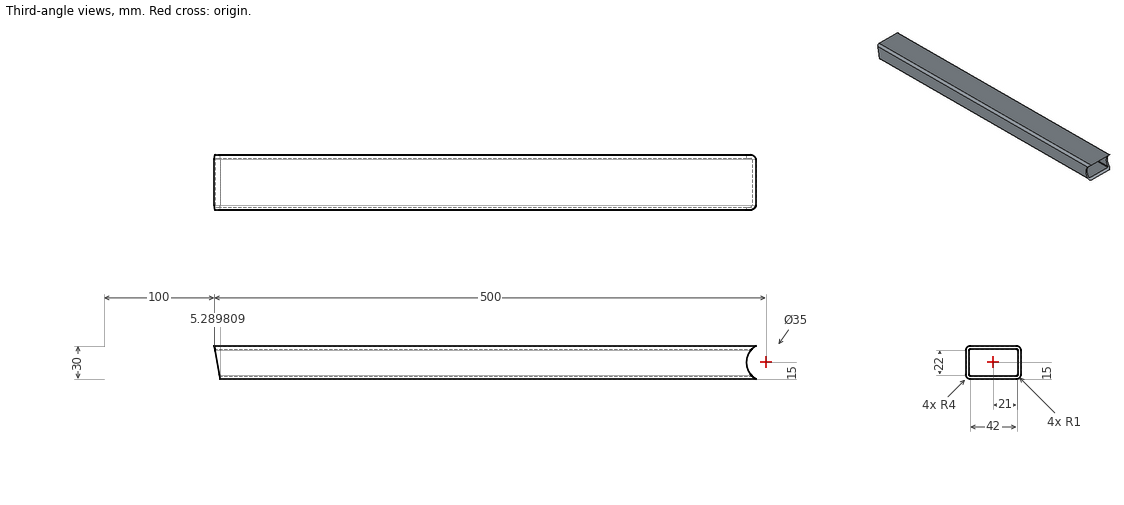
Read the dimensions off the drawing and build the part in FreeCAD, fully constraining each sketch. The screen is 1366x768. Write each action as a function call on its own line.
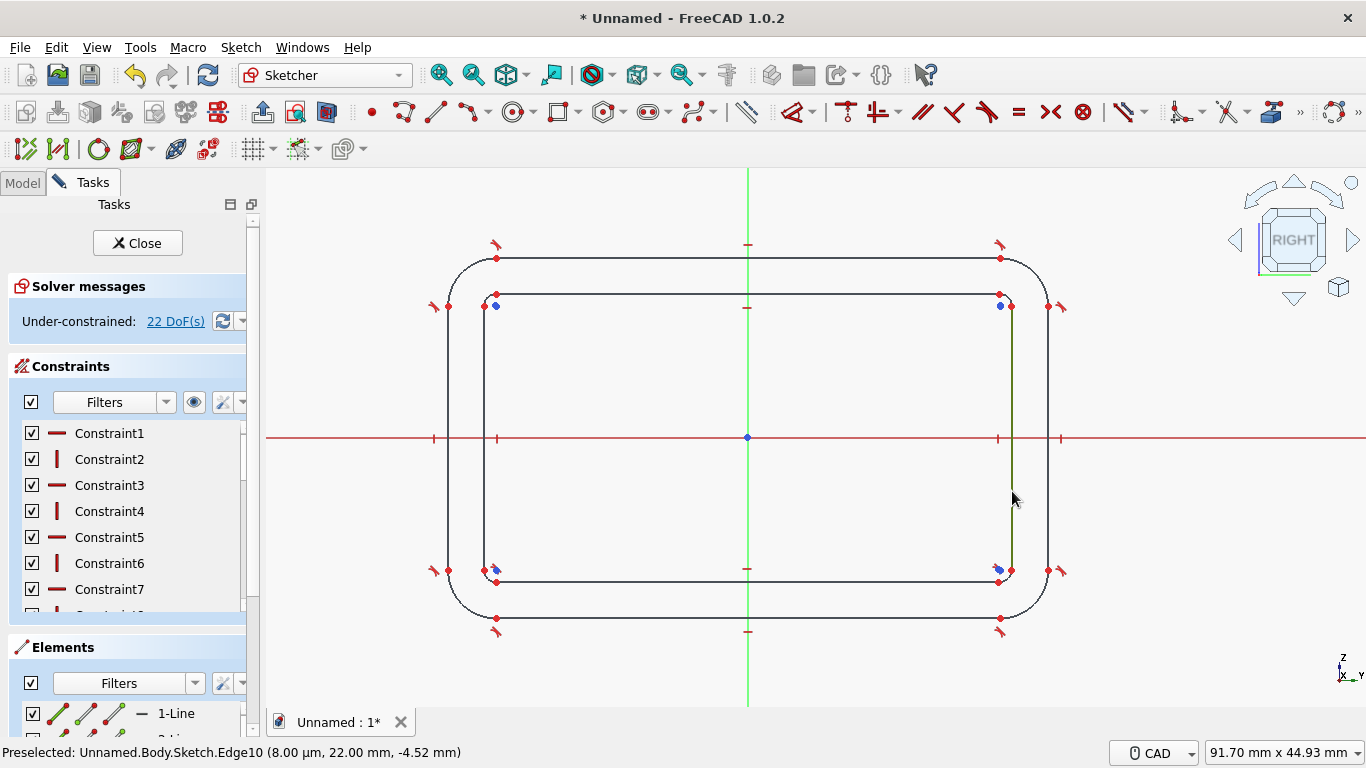
scroll(1008, 579, up, 2)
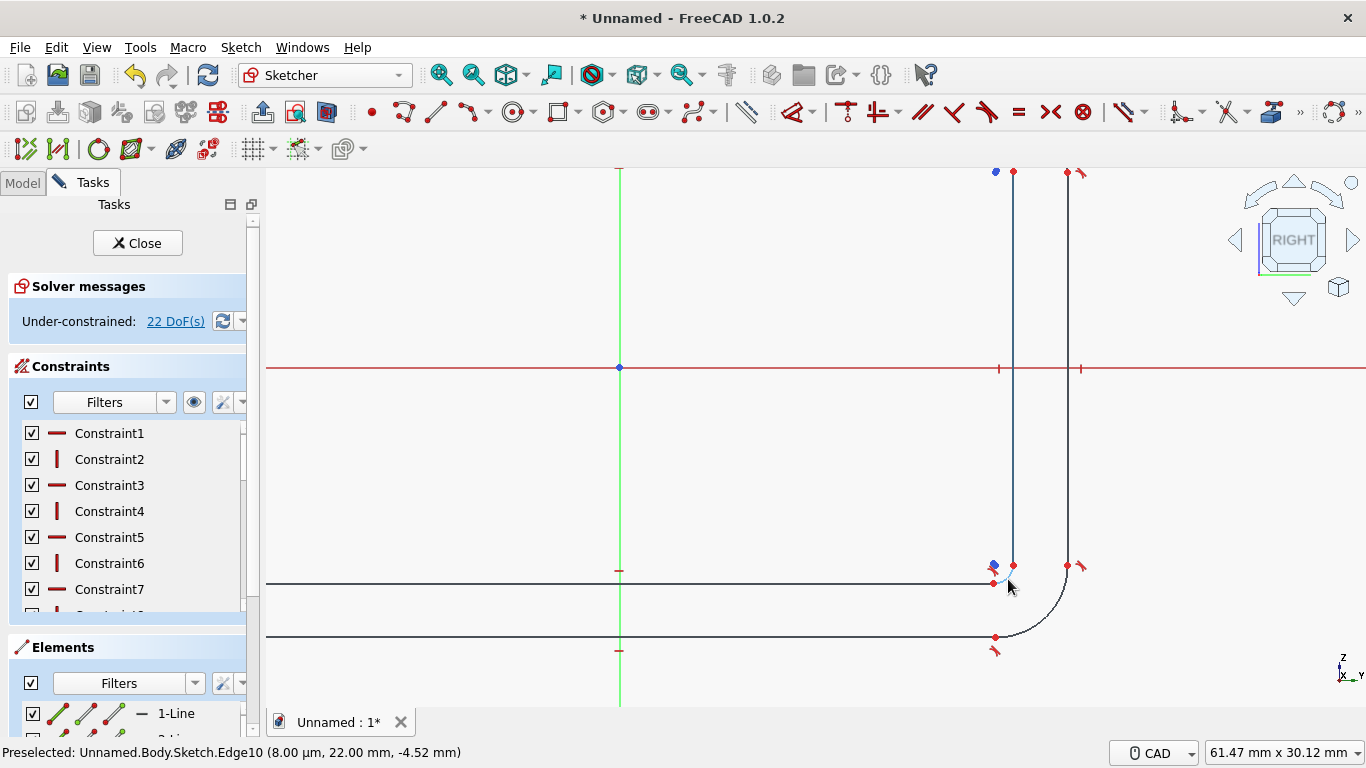
click(1007, 579)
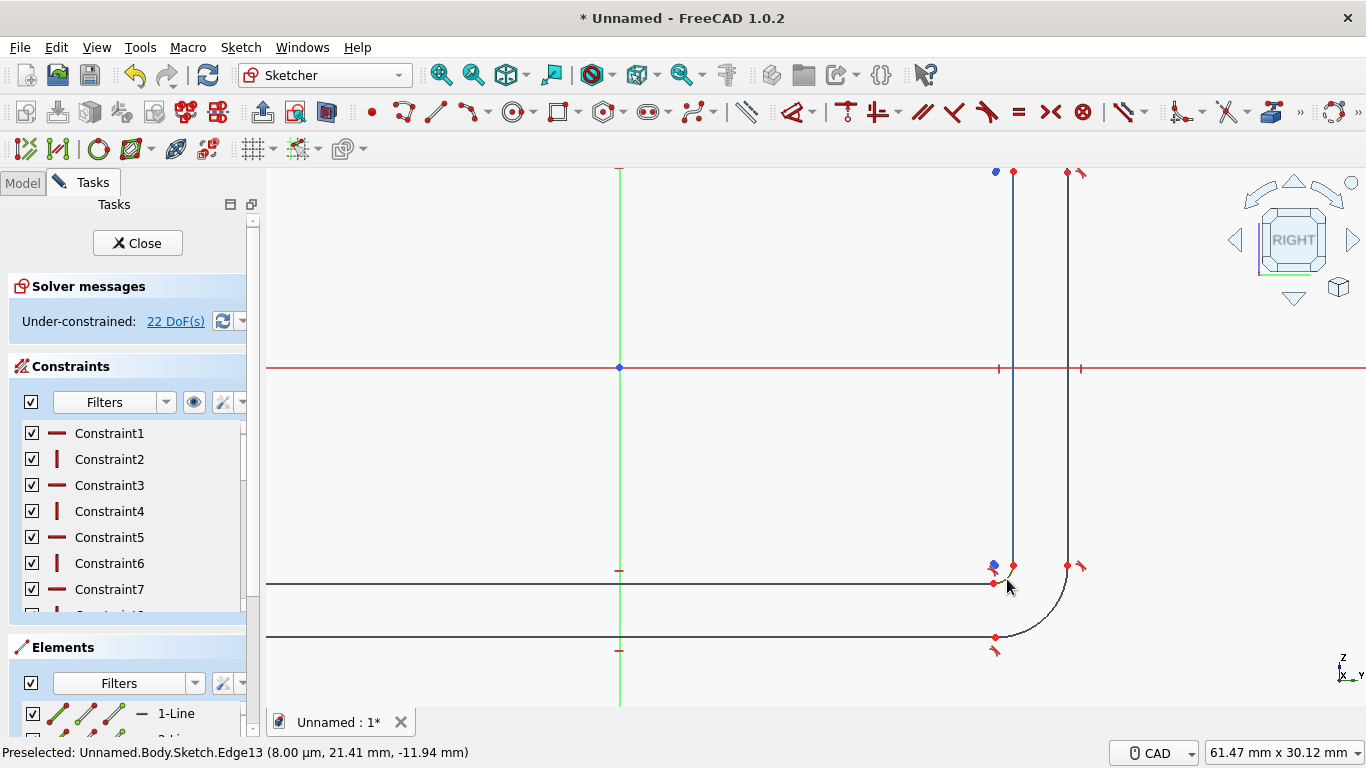
key(t)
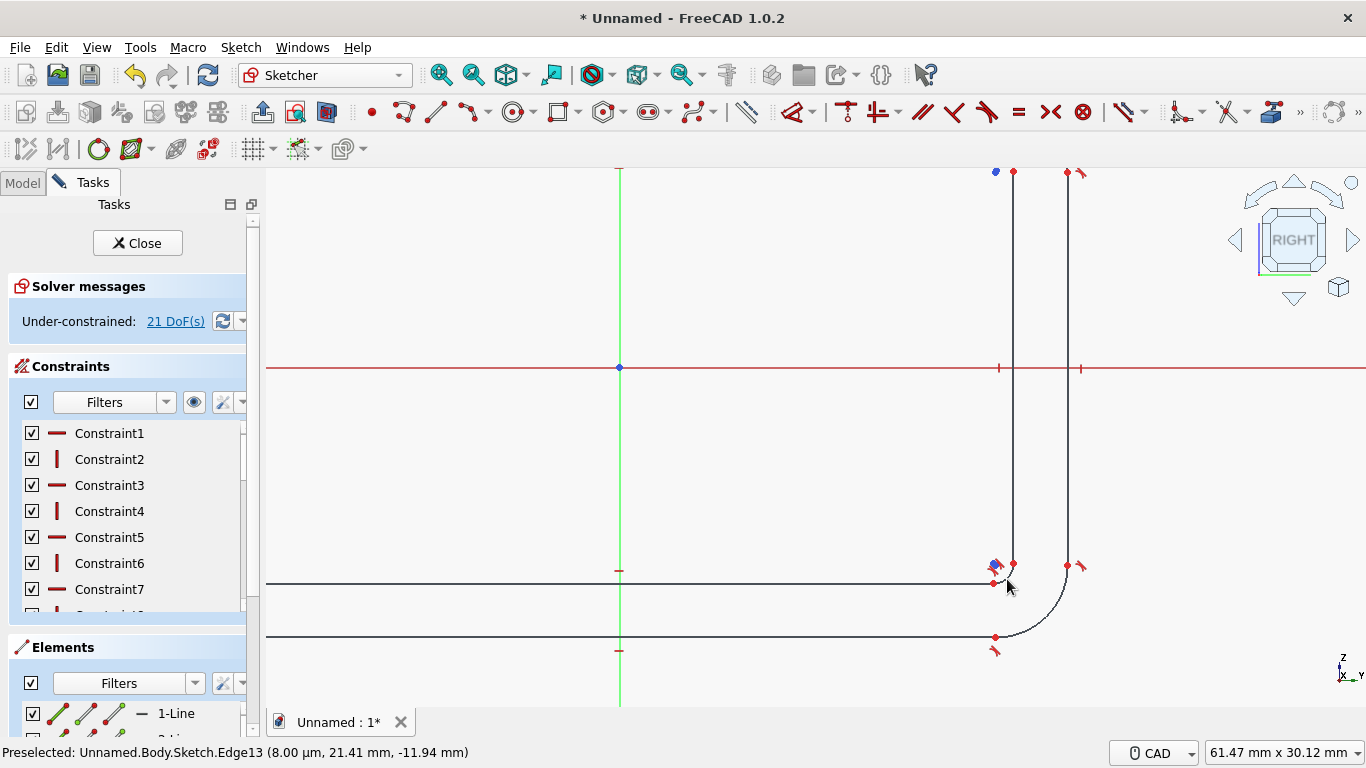
click(1013, 446)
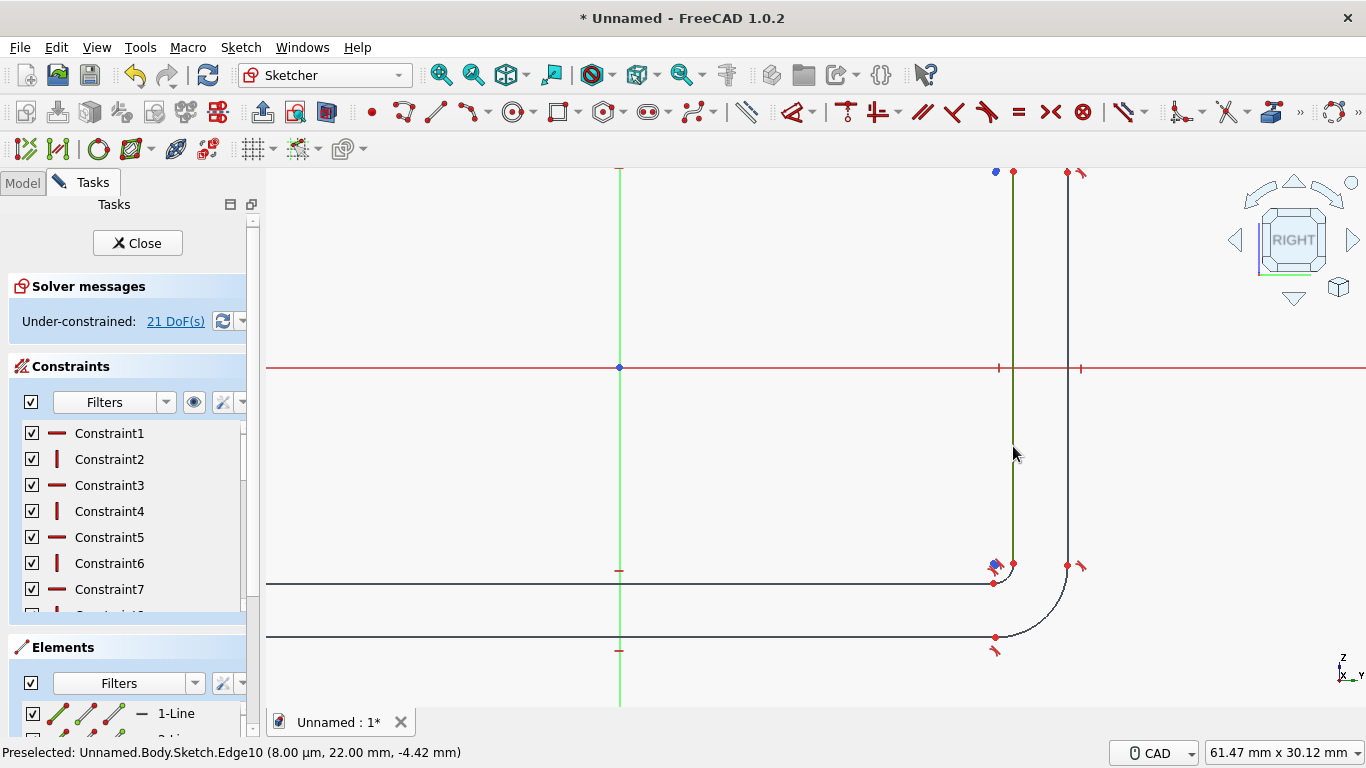
scroll(1008, 579, down, 2)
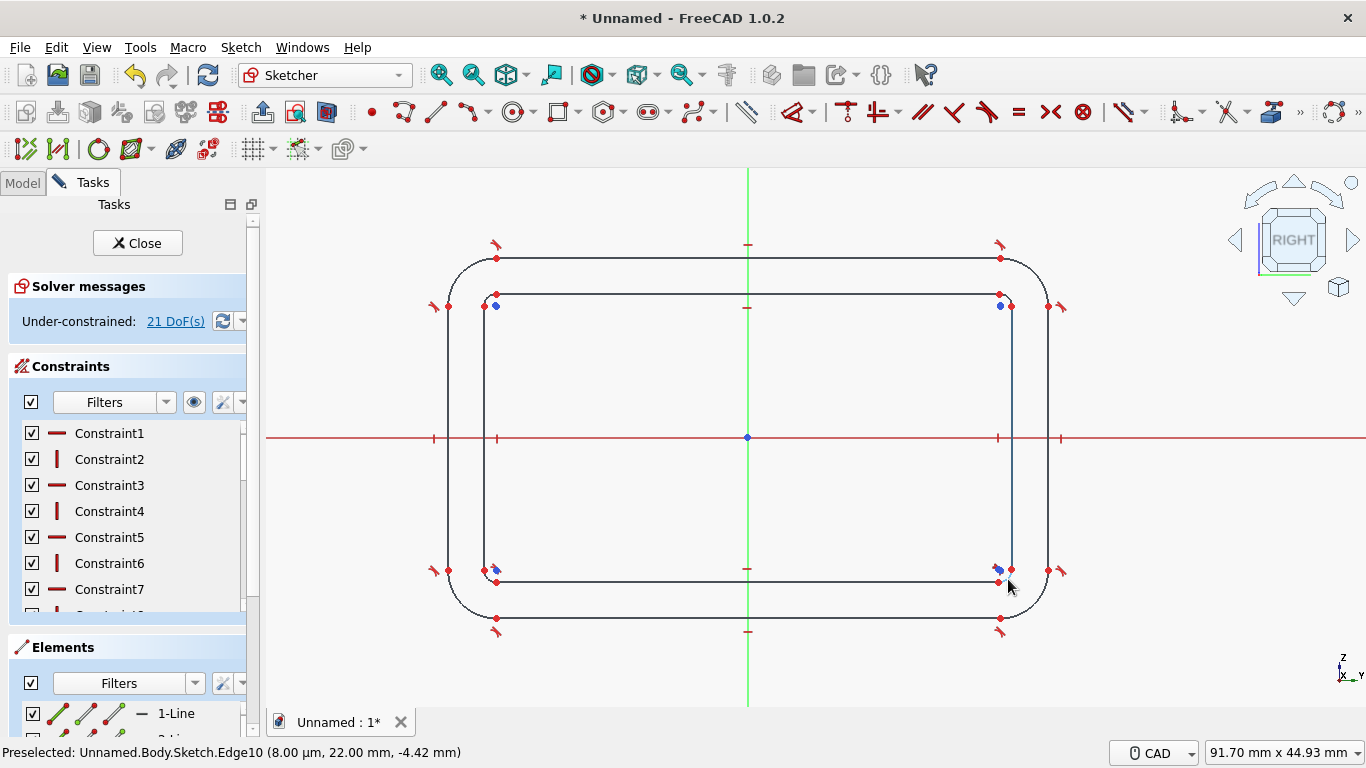
scroll(1008, 297, up, 2)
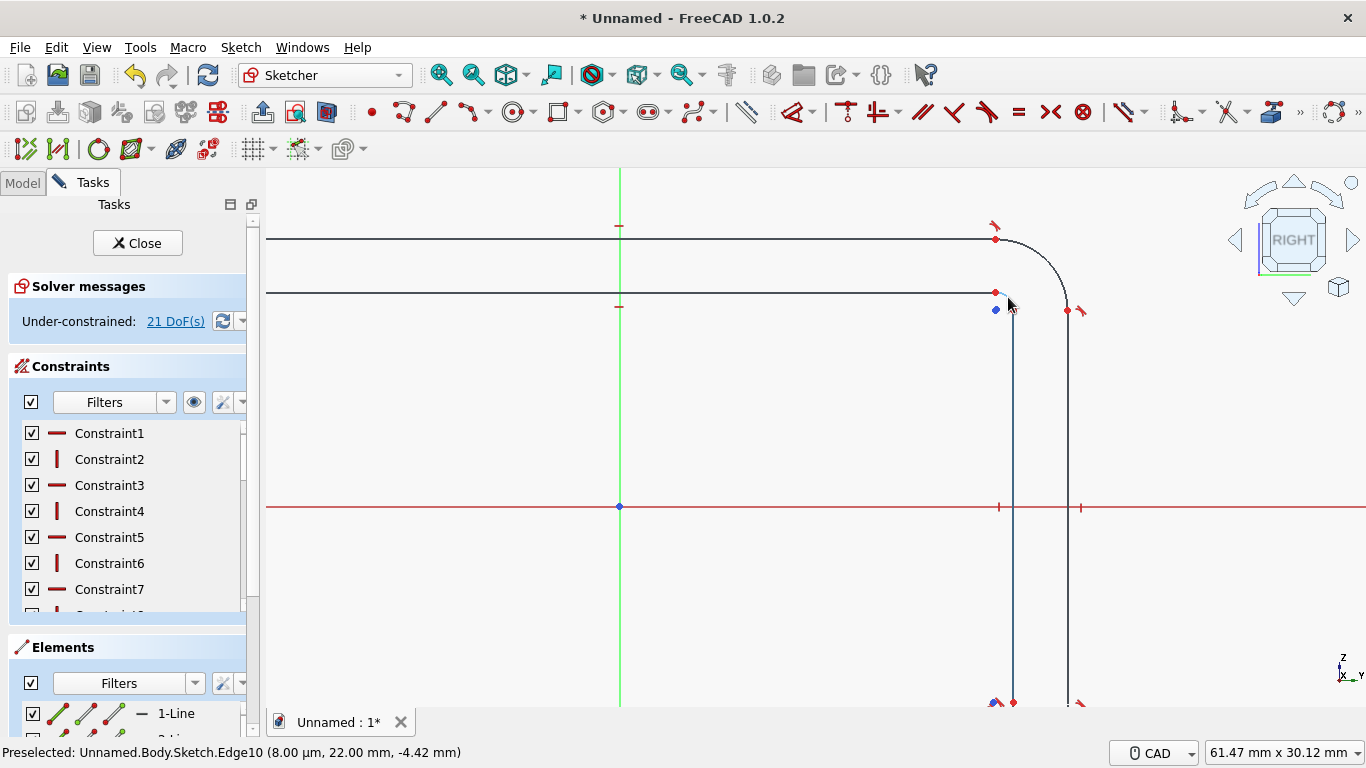
click(1008, 298)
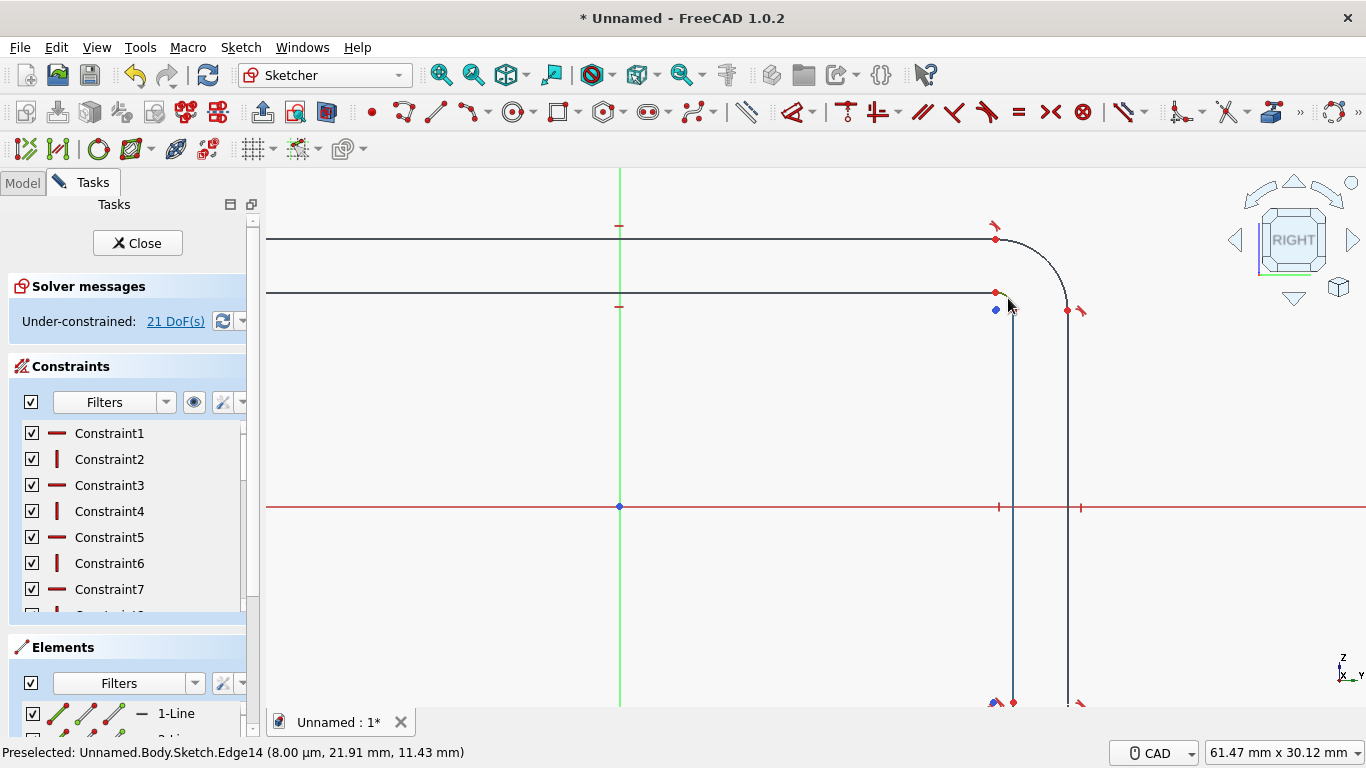
key(t)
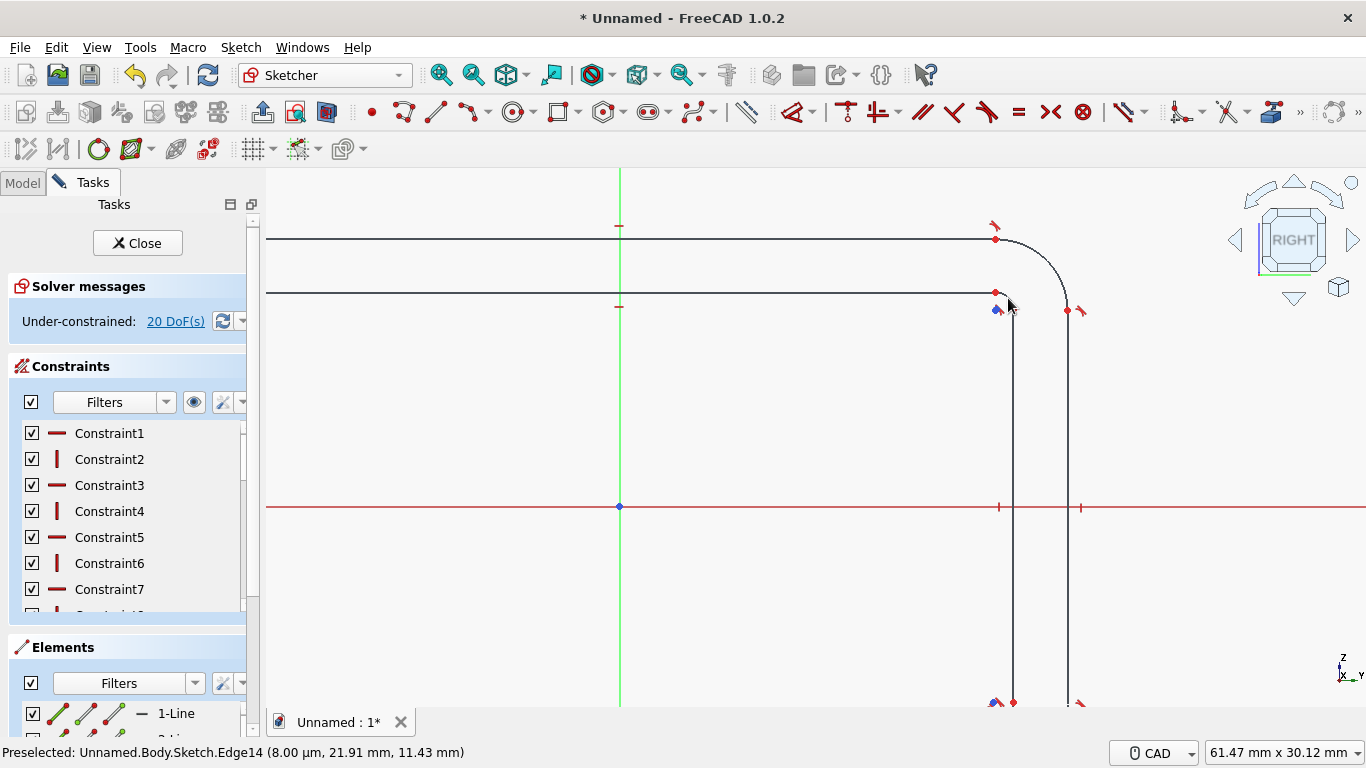
click(770, 293)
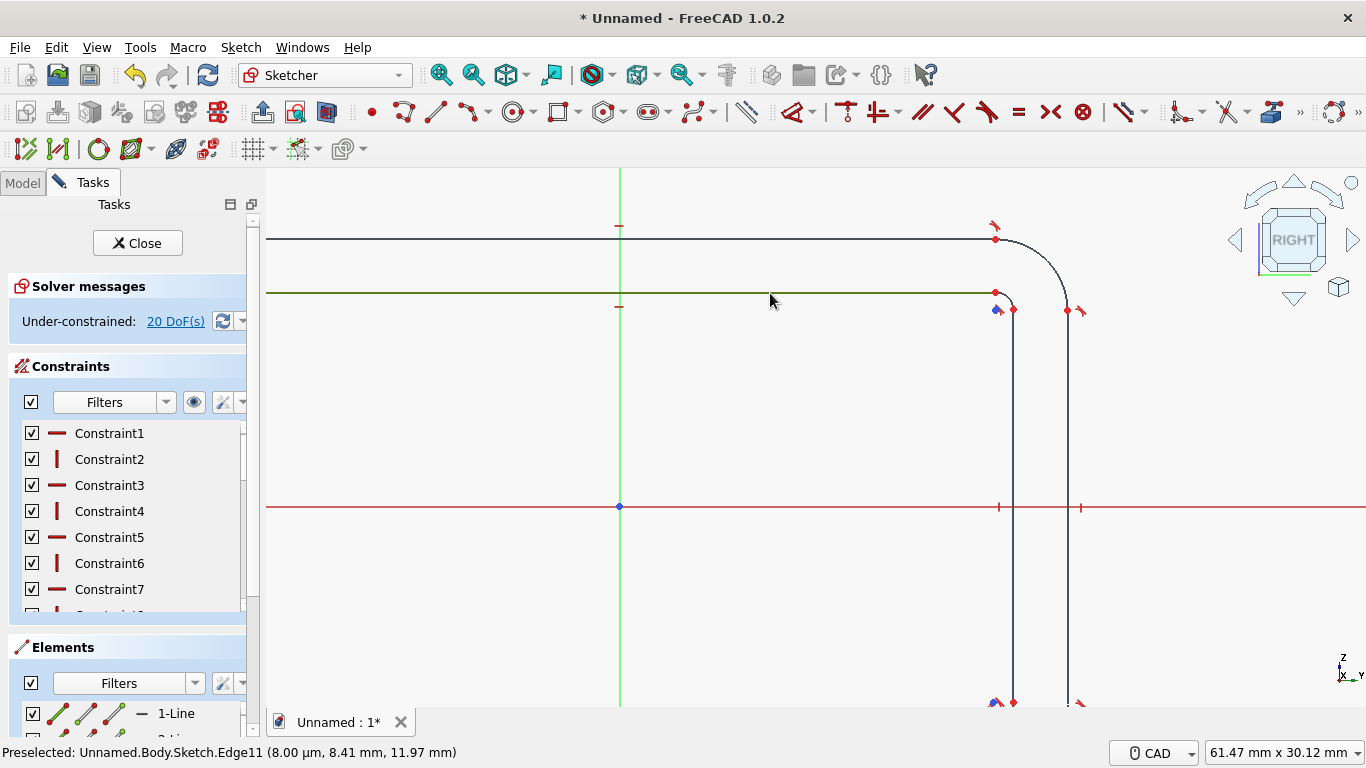
click(1008, 297)